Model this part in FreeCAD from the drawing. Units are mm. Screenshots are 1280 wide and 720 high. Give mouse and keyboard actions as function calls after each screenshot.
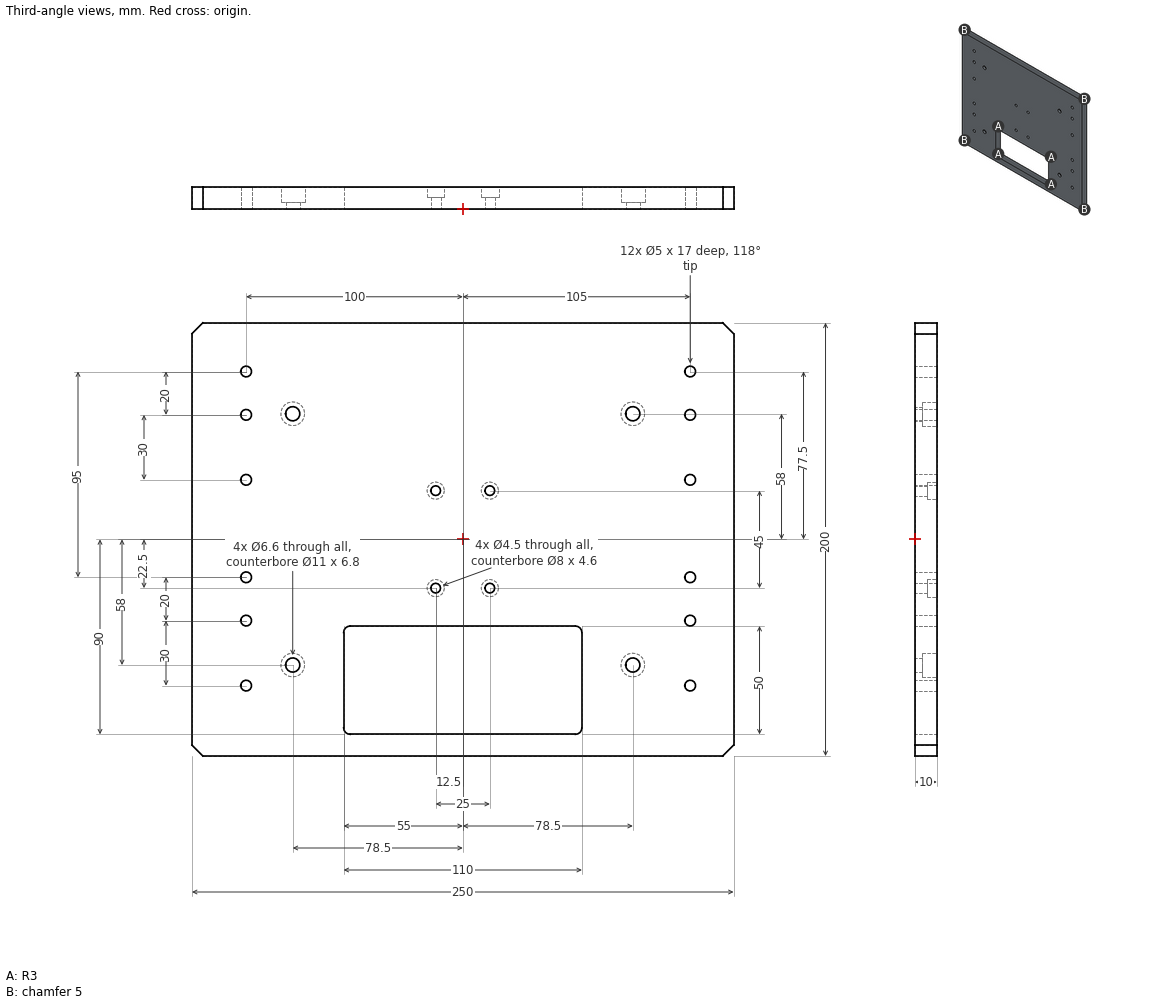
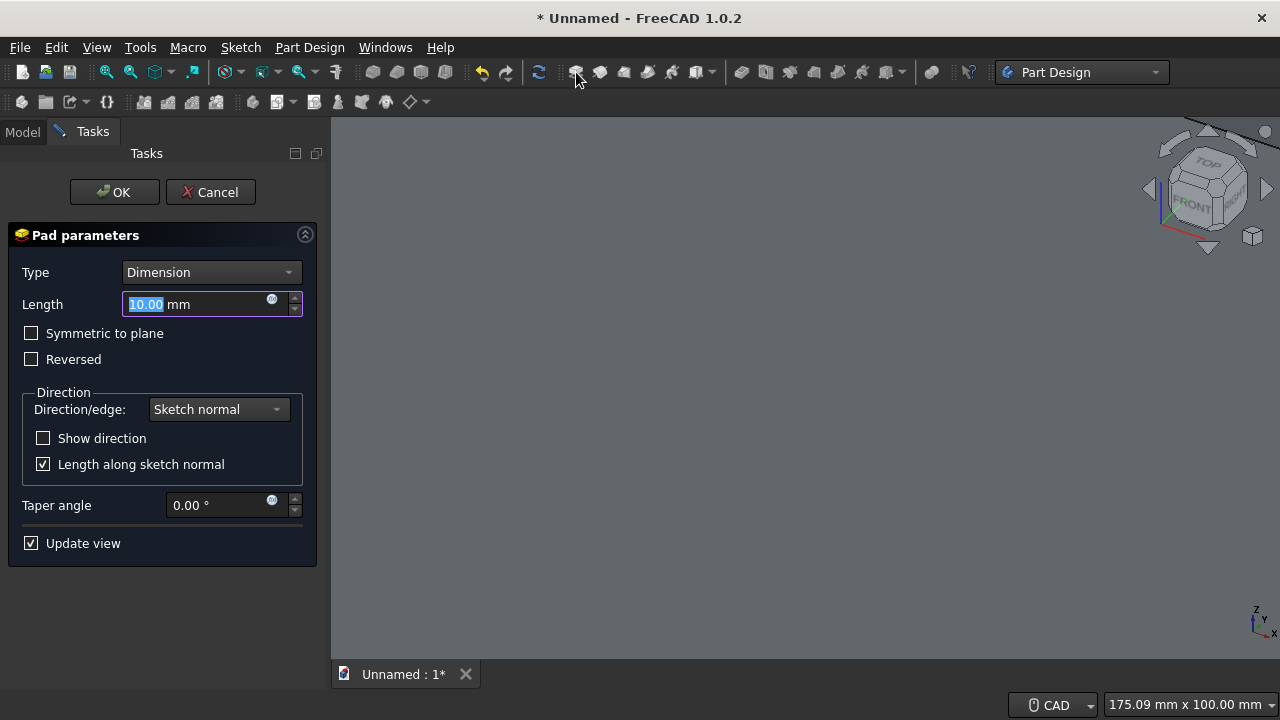
text(10)
key(Tab)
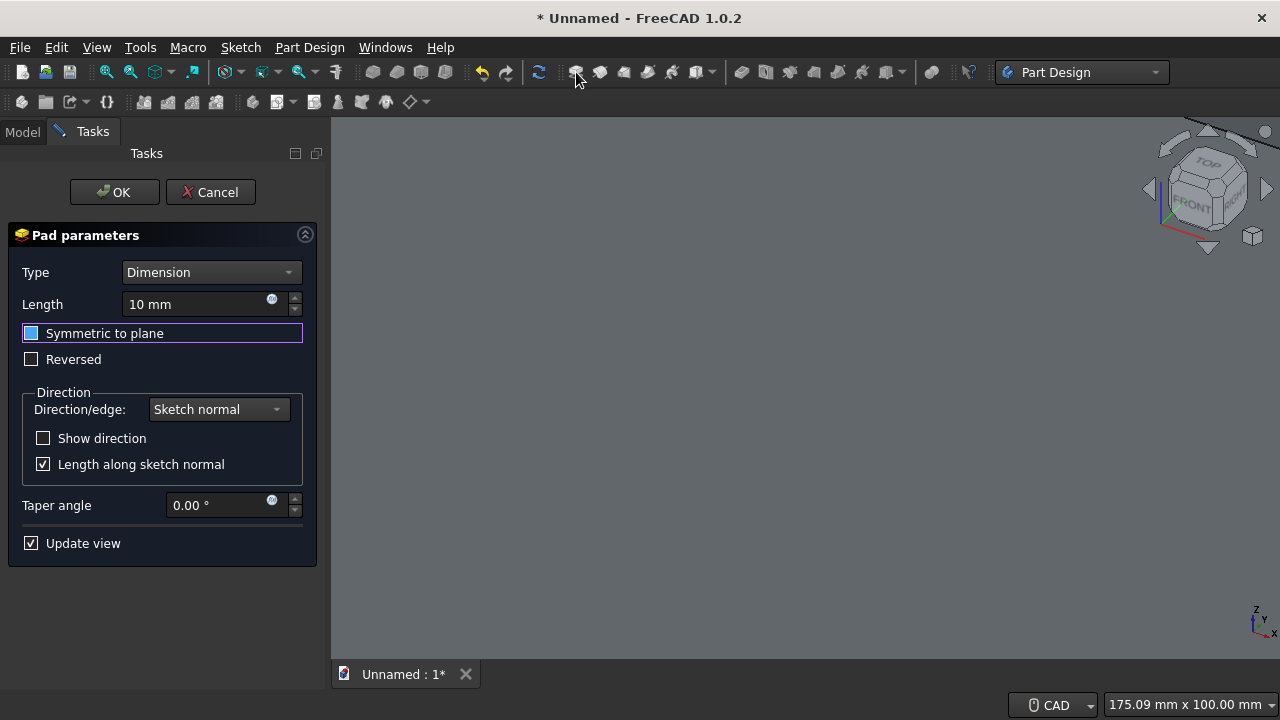
click(30, 359)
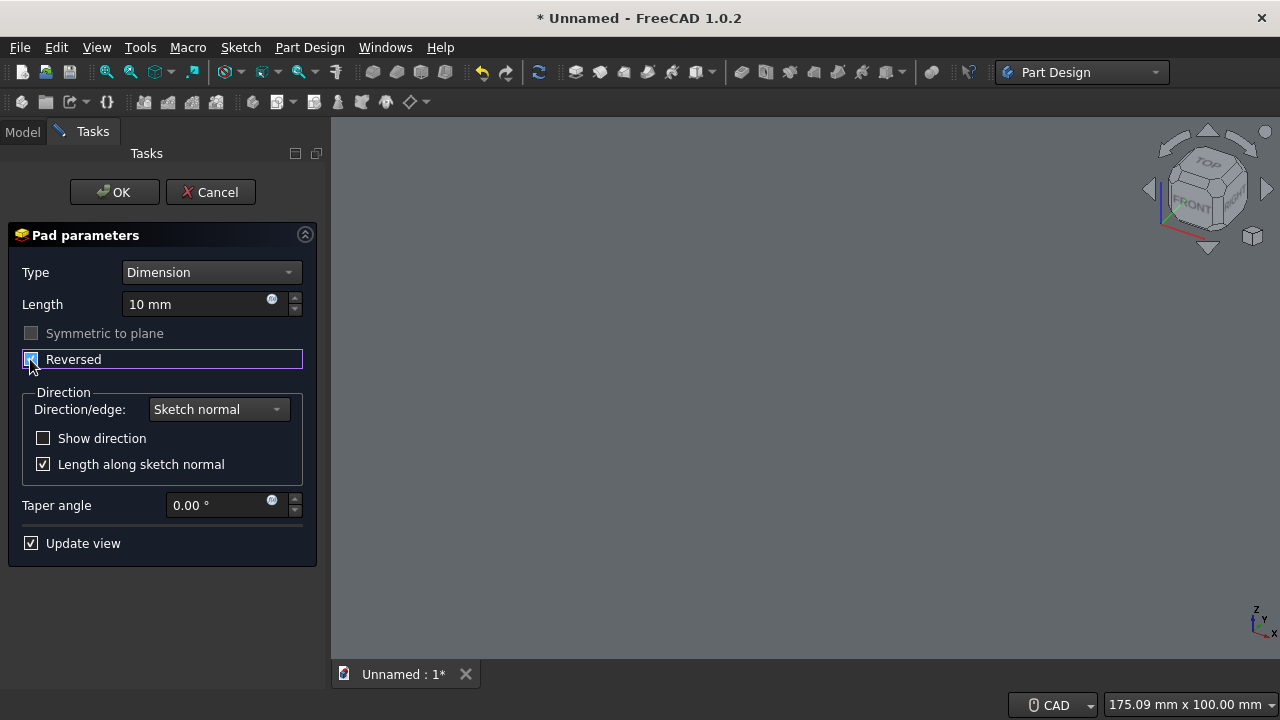
click(115, 192)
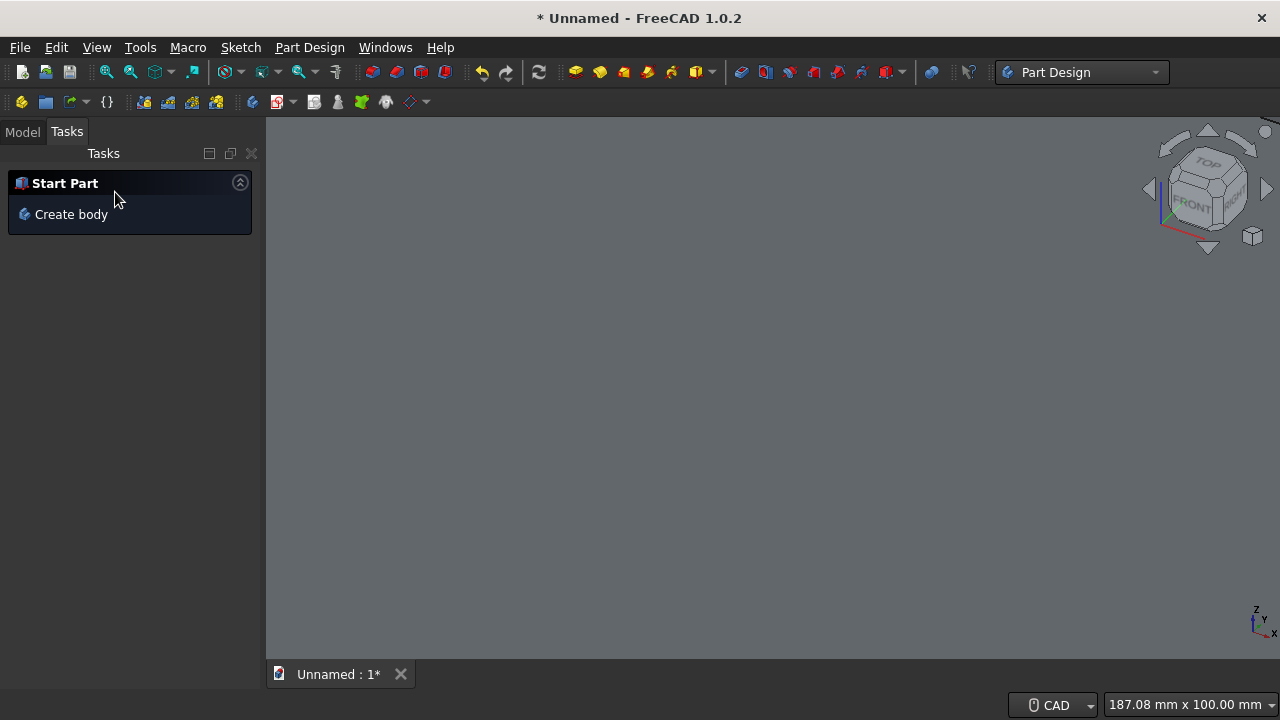
click(108, 72)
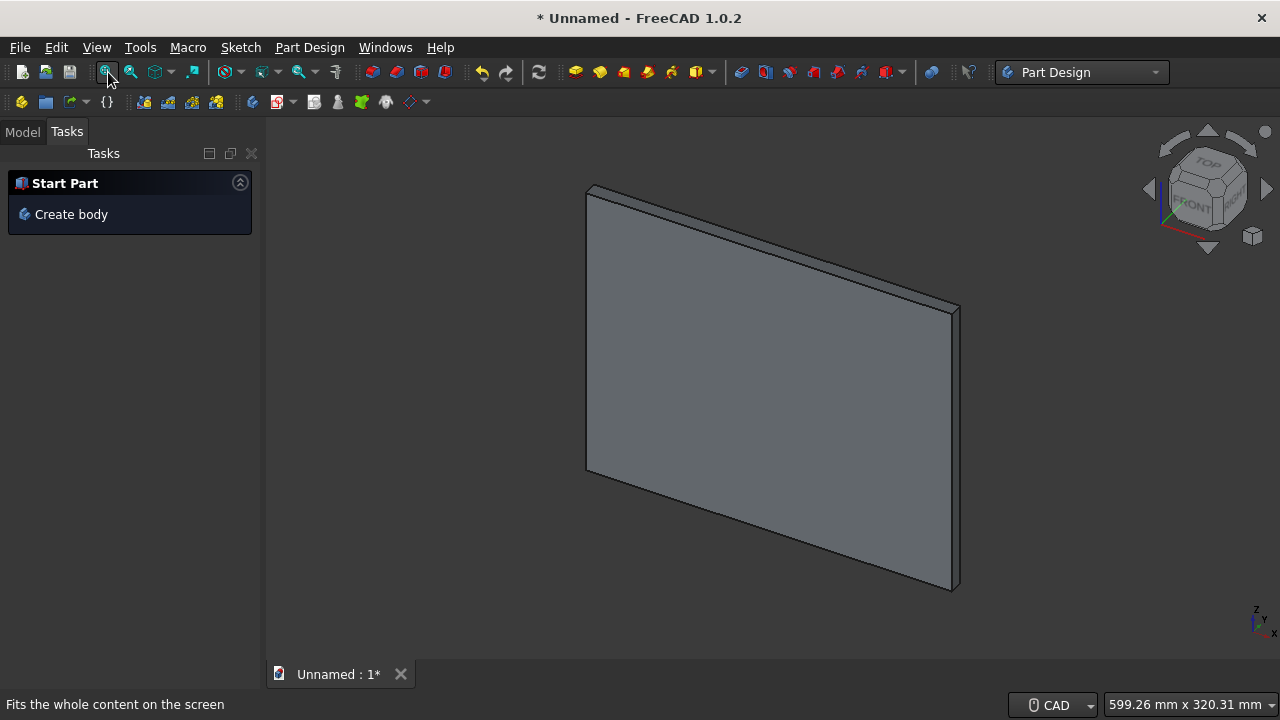
key(4)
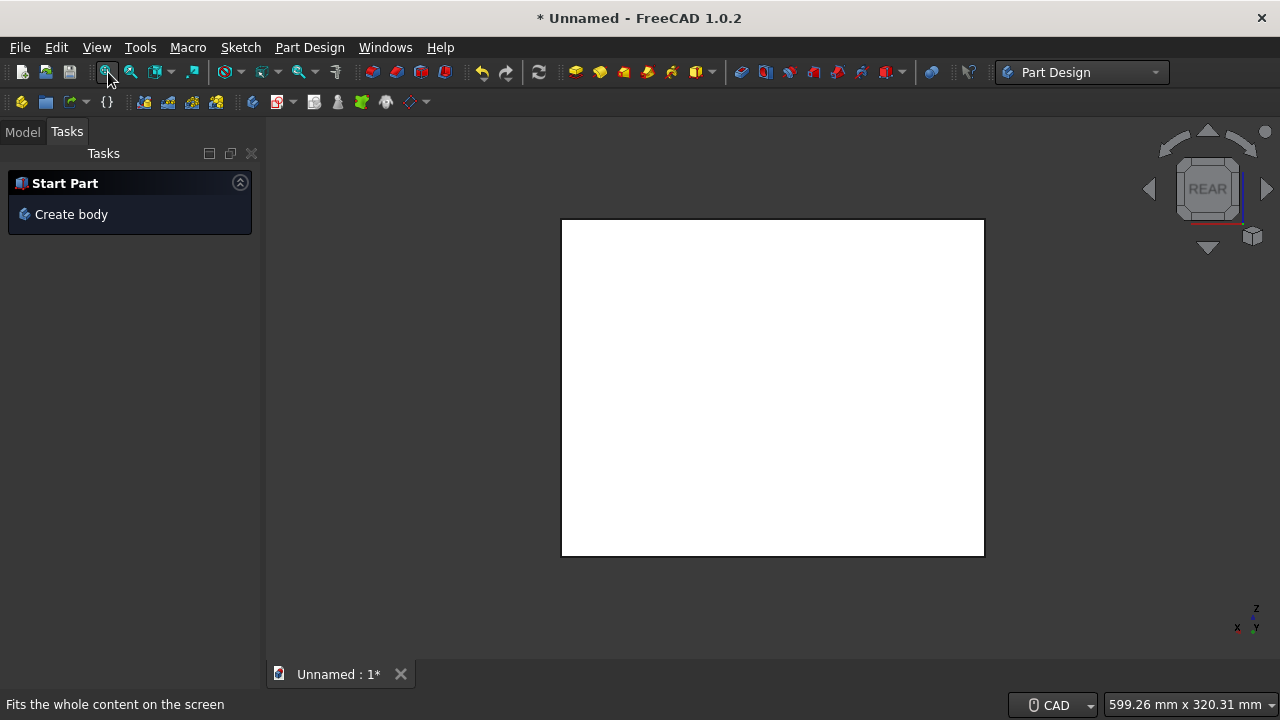
click(773, 387)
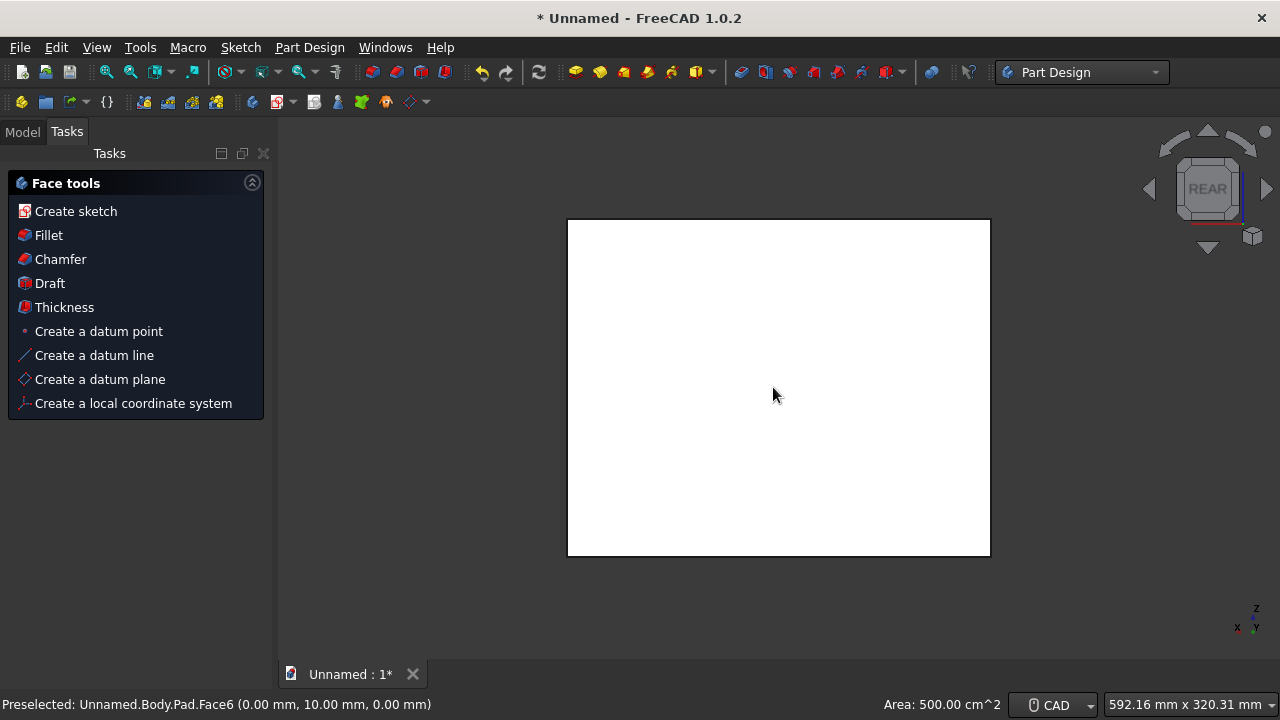
click(278, 102)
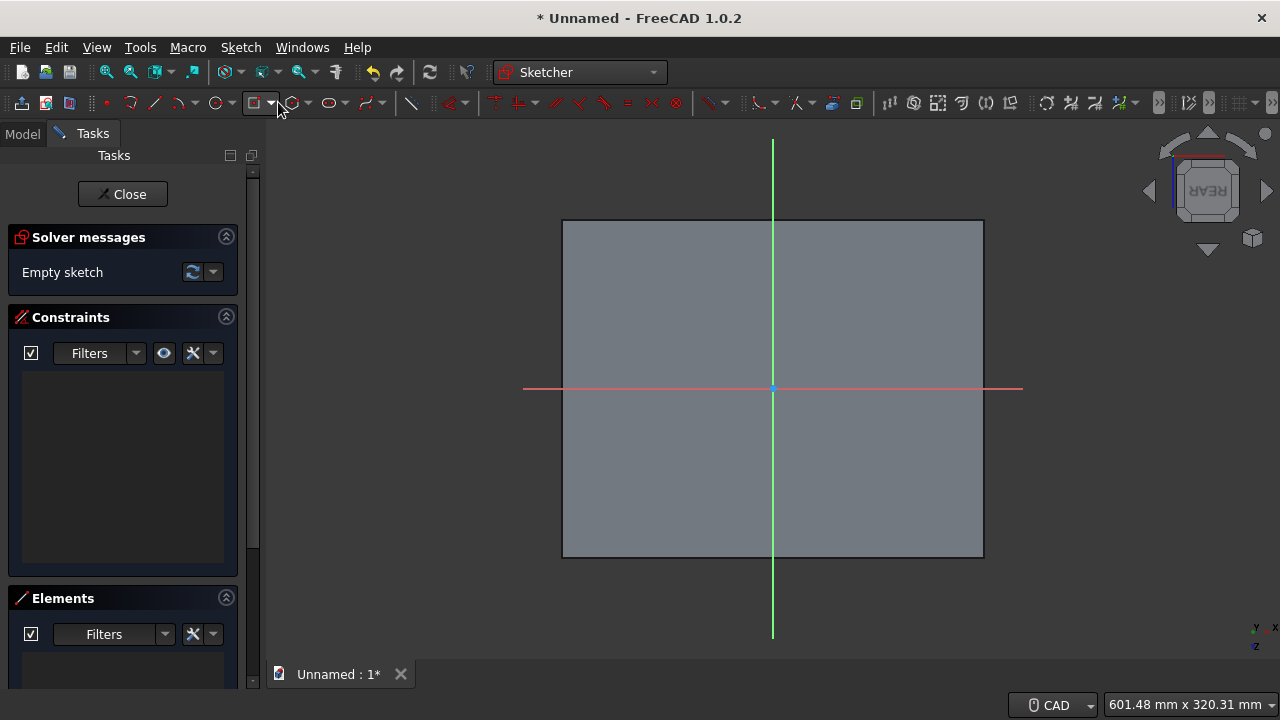
scroll(925, 415, up, 2)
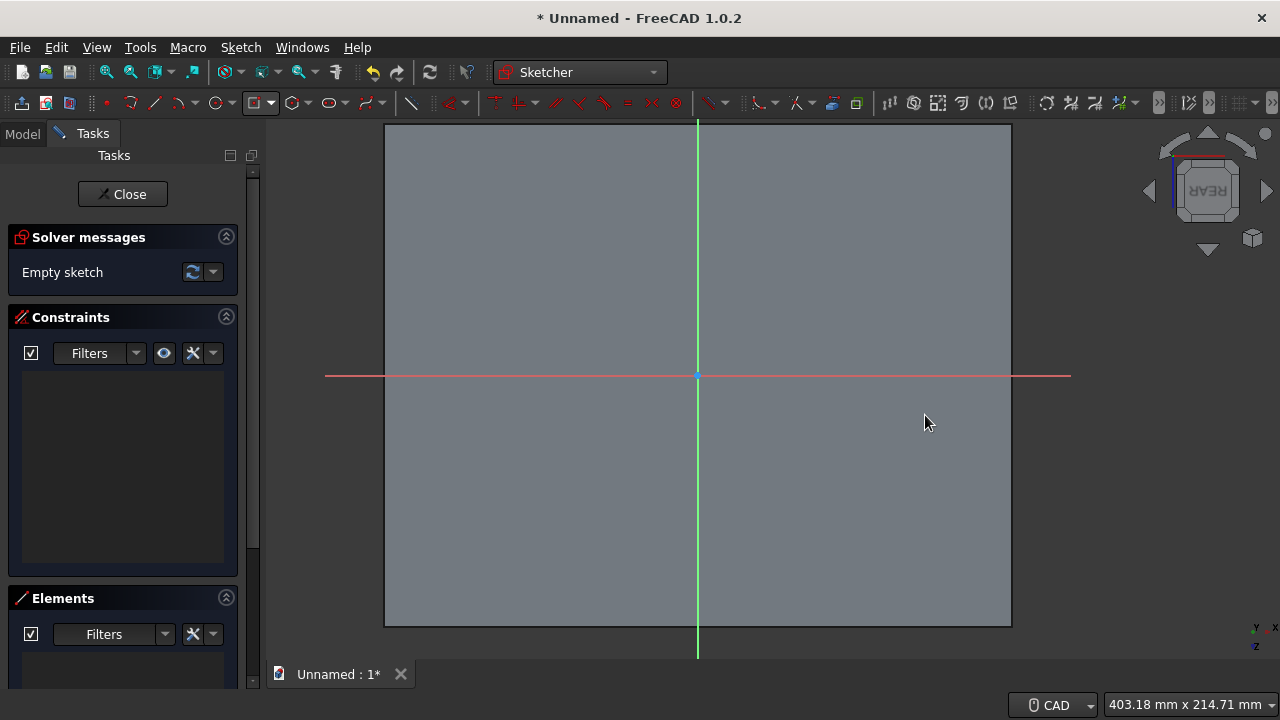
click(216, 104)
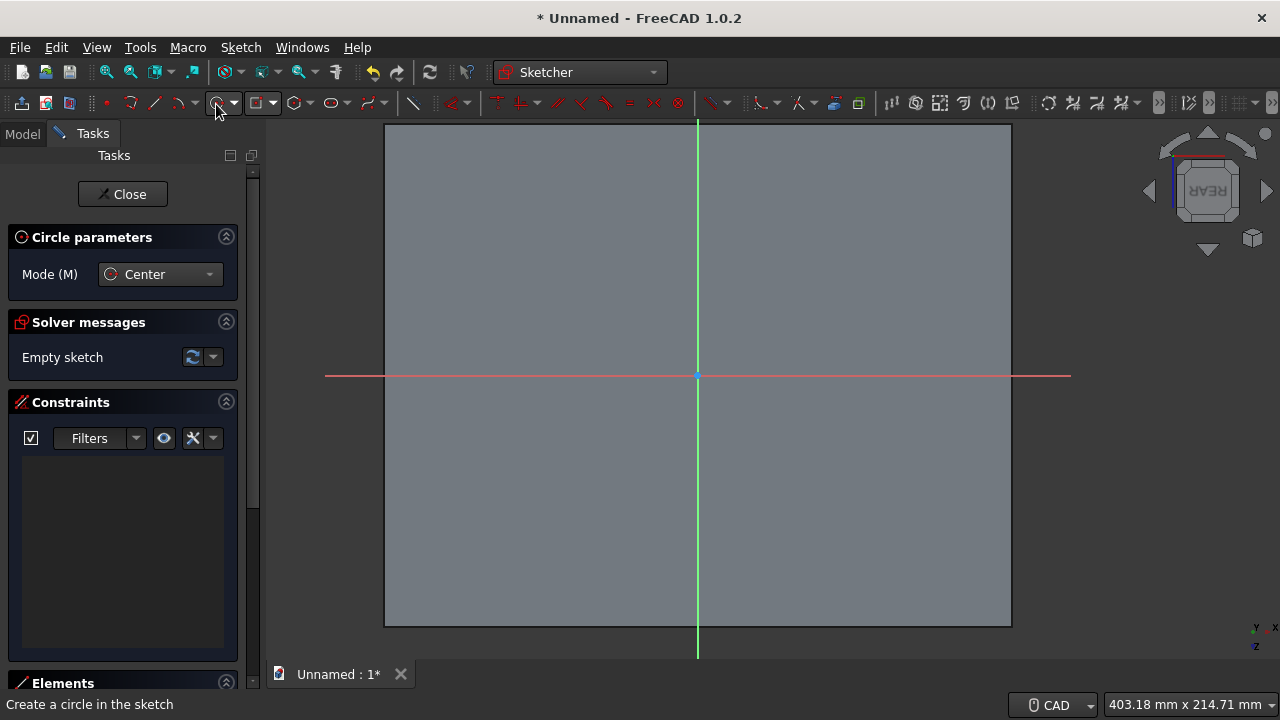
scroll(962, 571, up, 7)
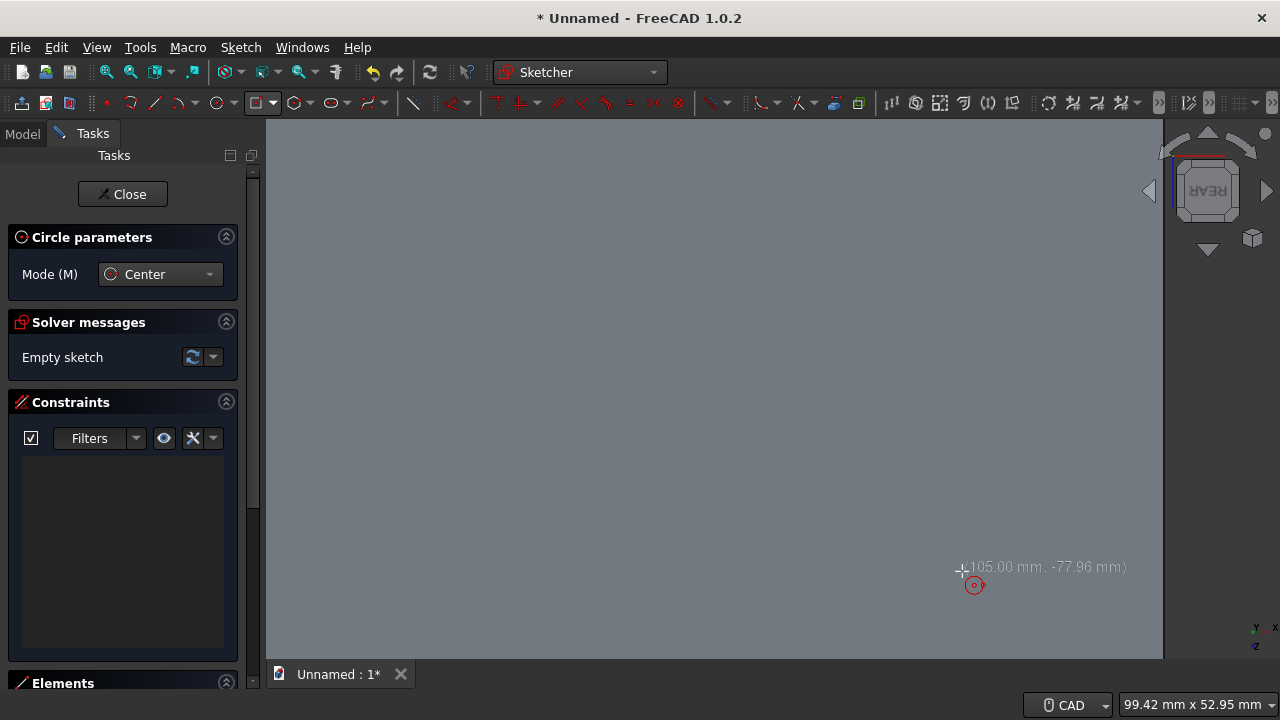
scroll(963, 572, down, 7)